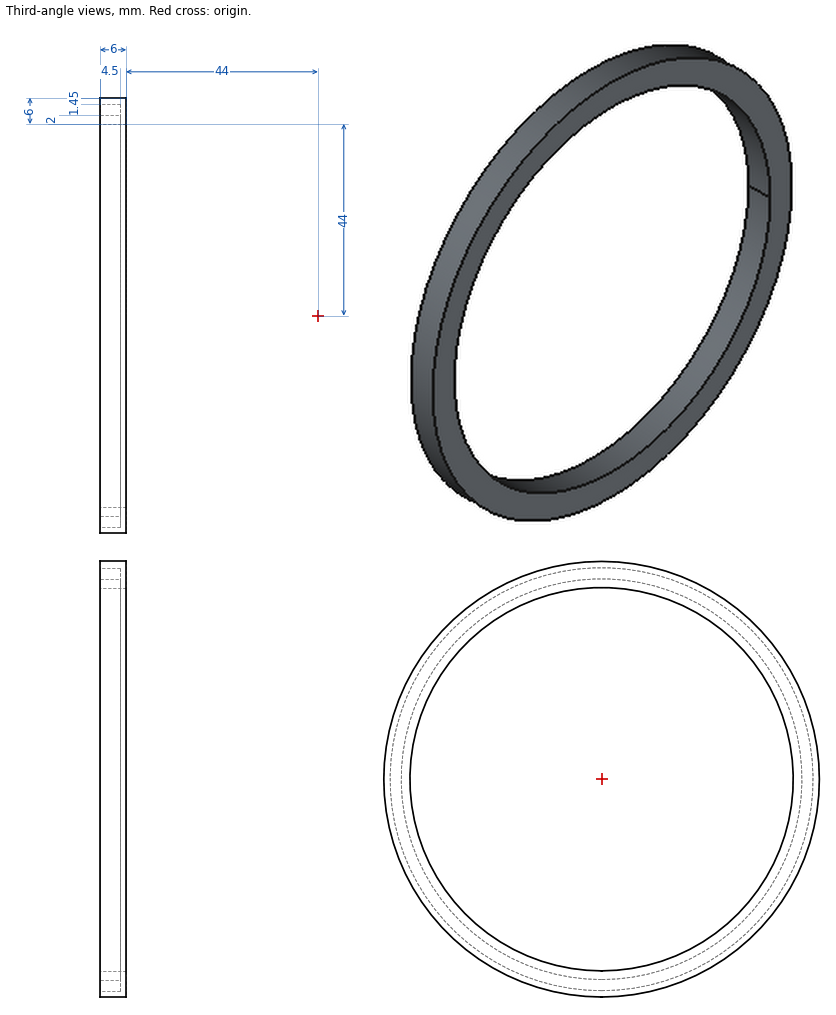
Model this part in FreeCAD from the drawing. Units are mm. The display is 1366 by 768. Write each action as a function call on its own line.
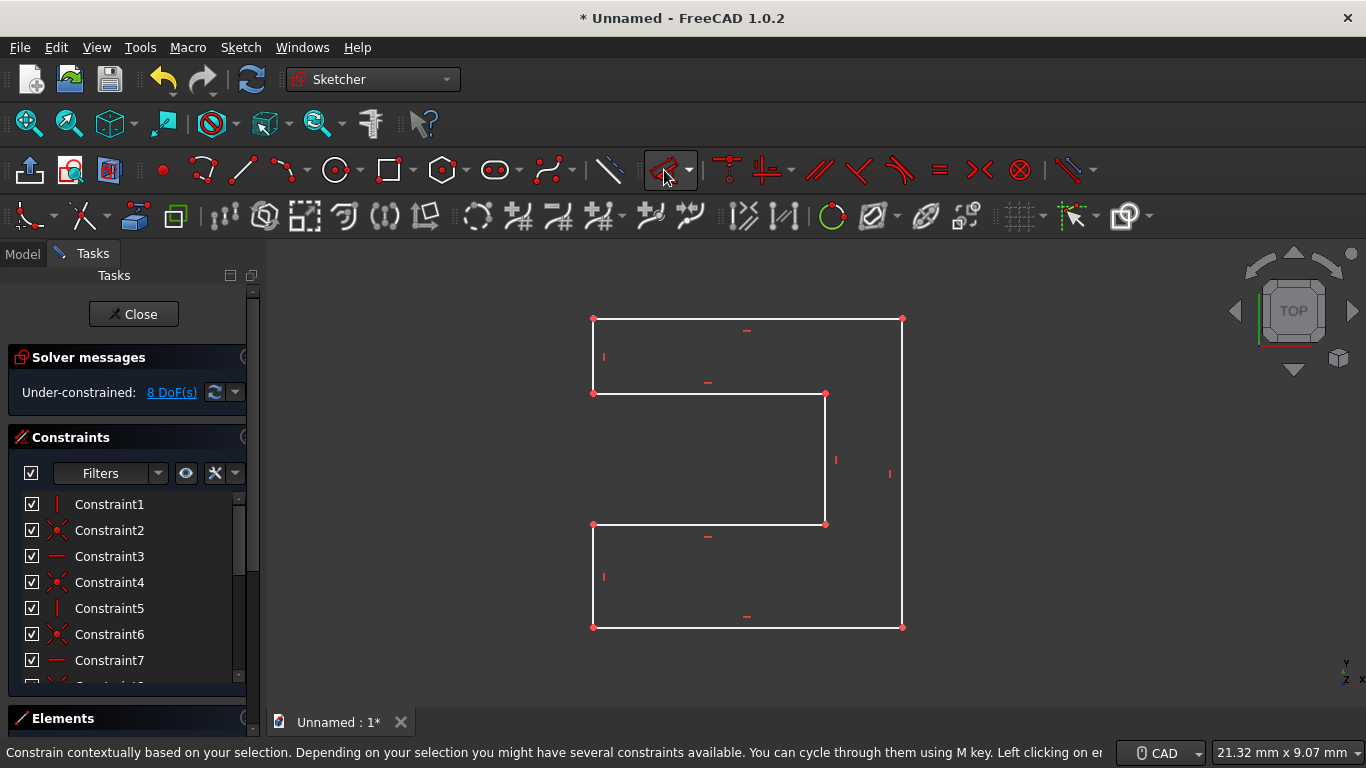
click(902, 535)
click(936, 473)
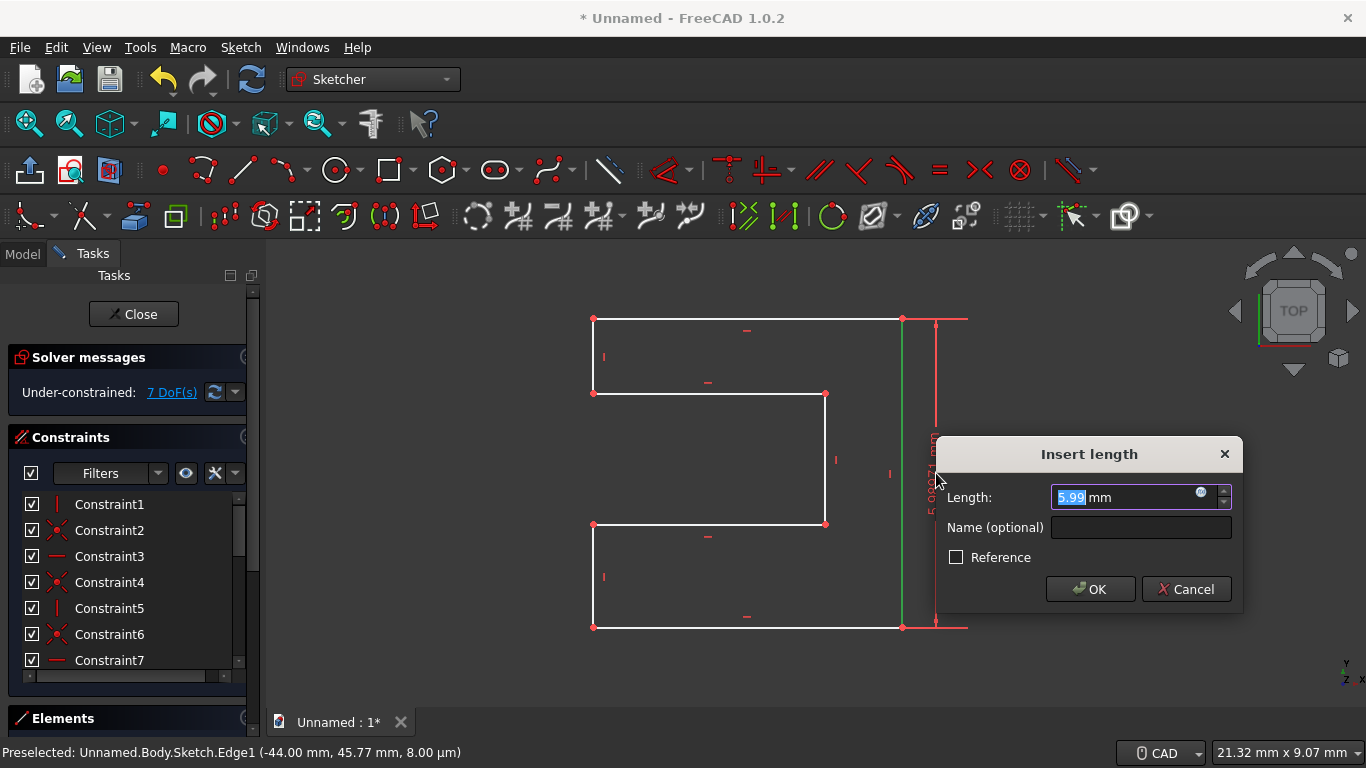
text(6)
key(Return)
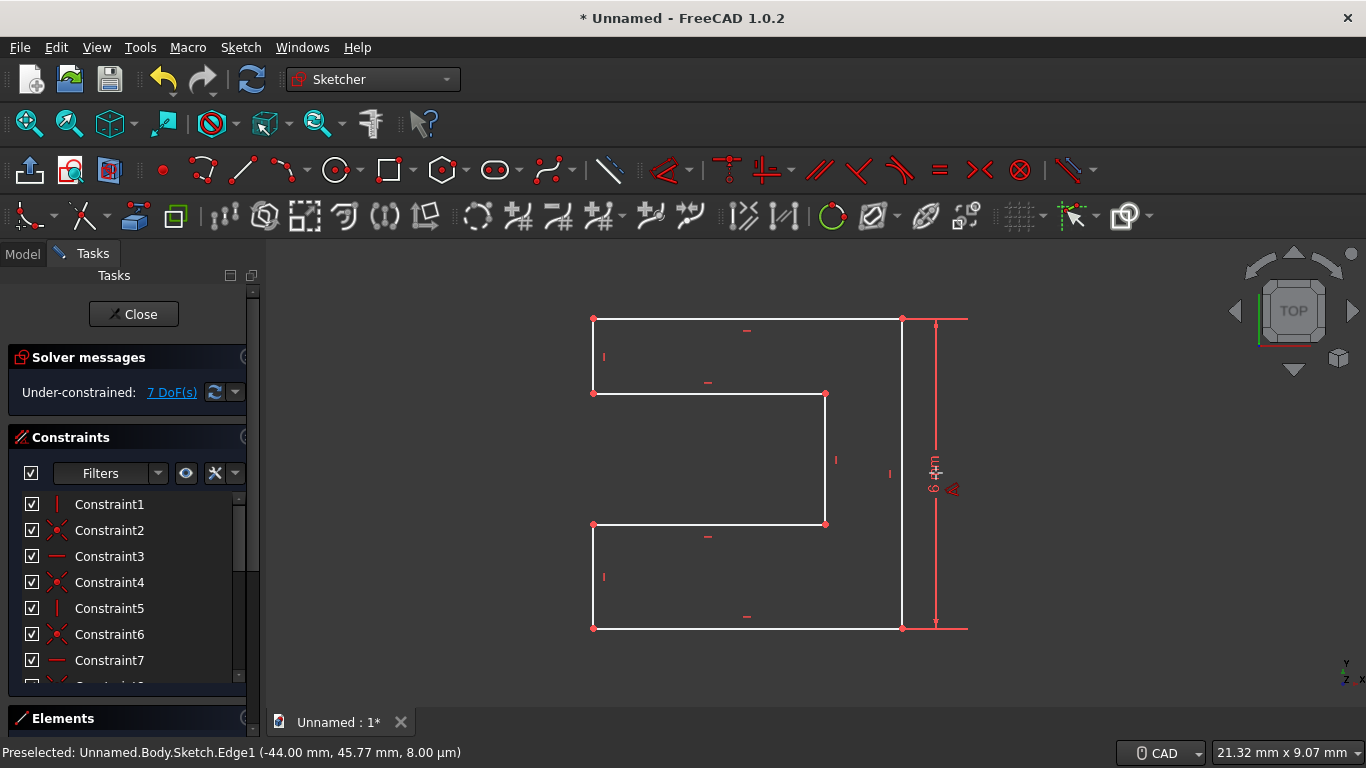
click(809, 319)
click(747, 285)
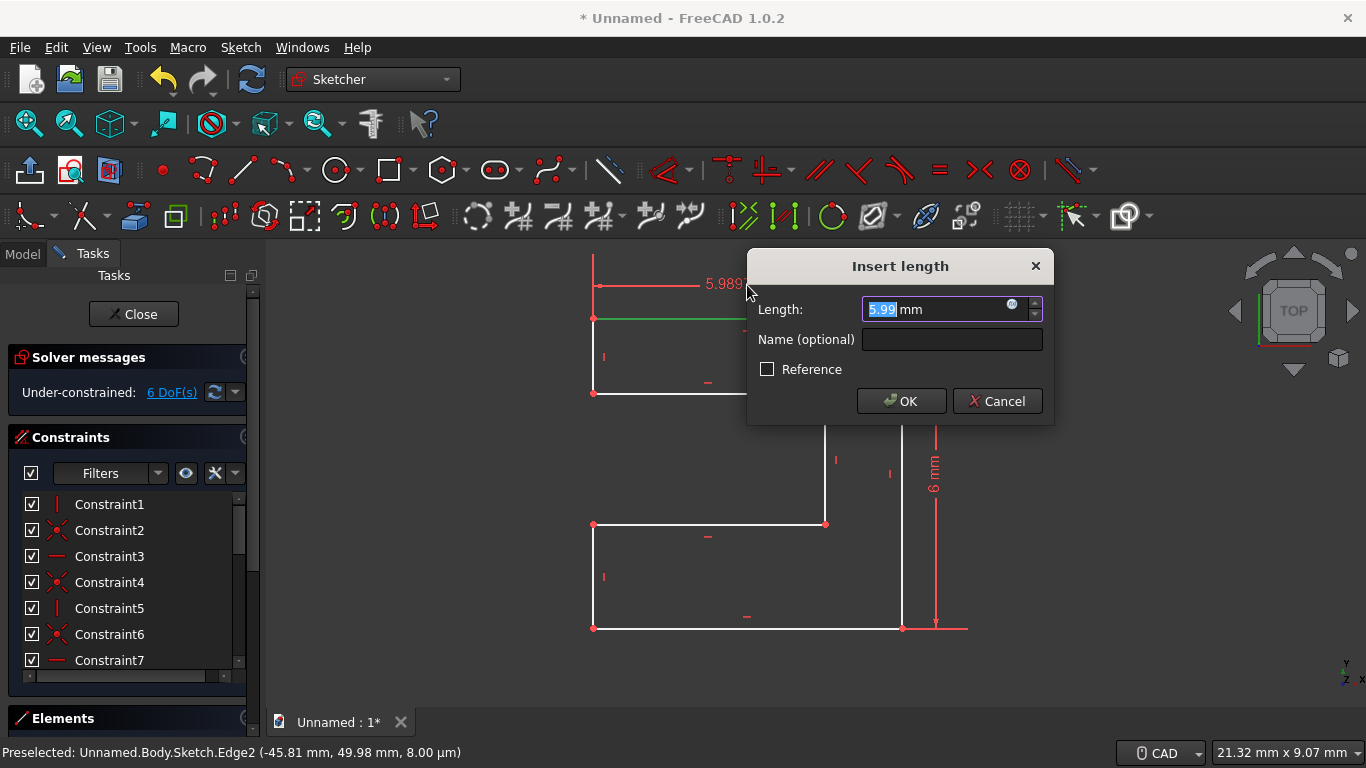
text(6)
key(Return)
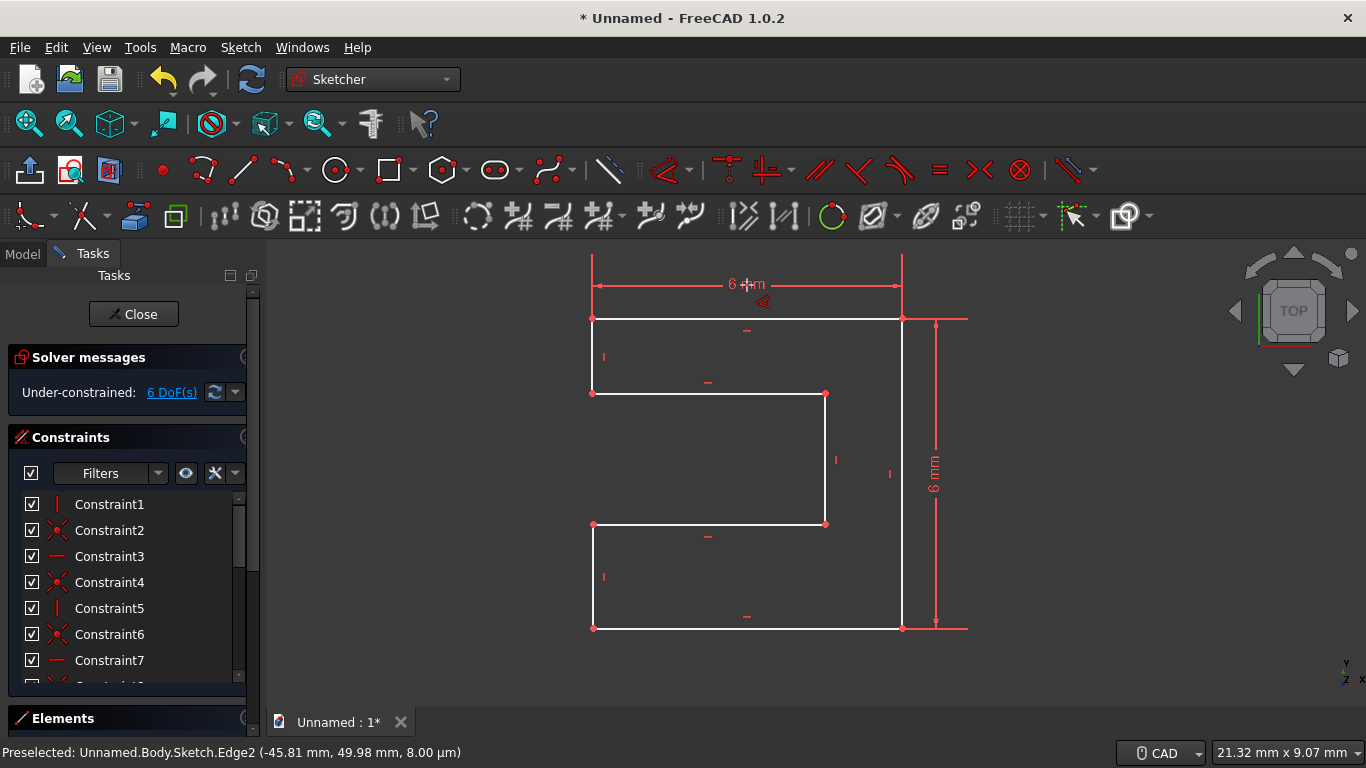
click(593, 556)
click(559, 577)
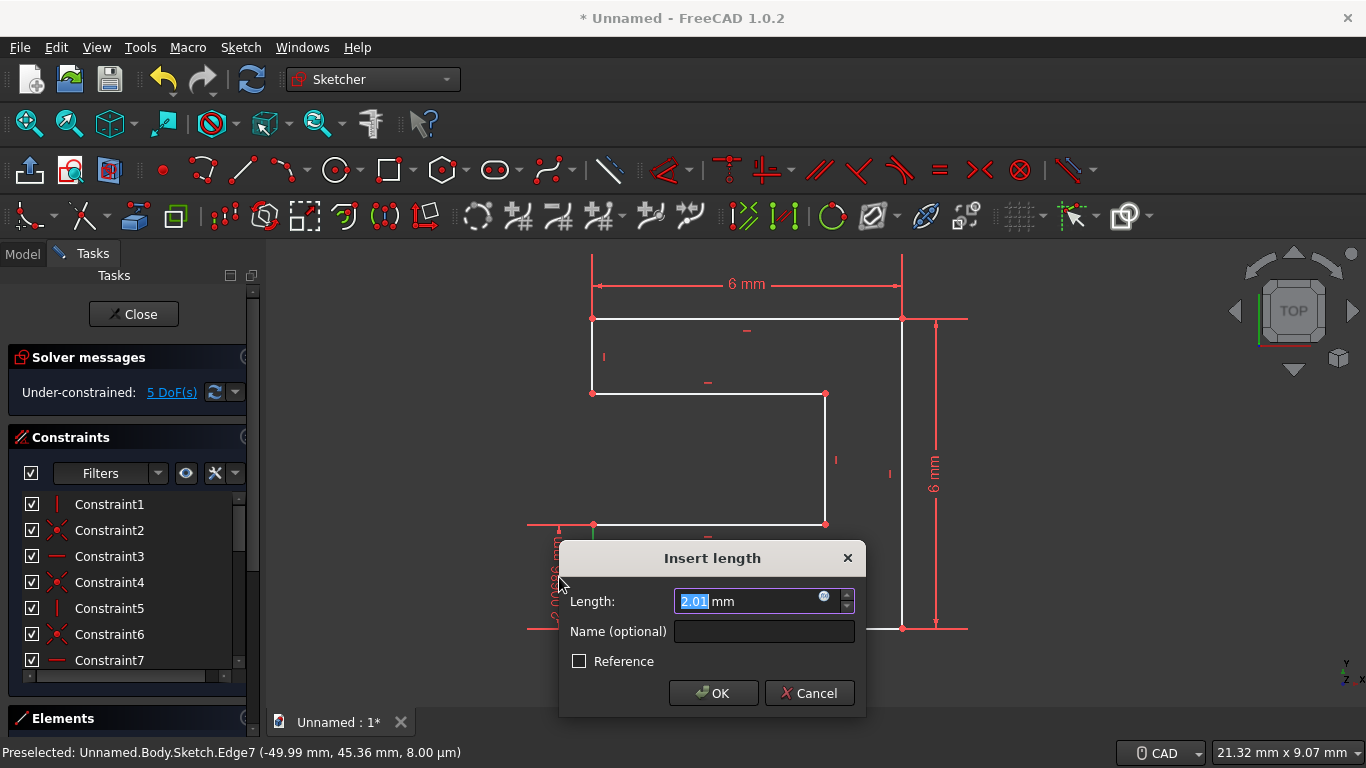
text(2)
key(Return)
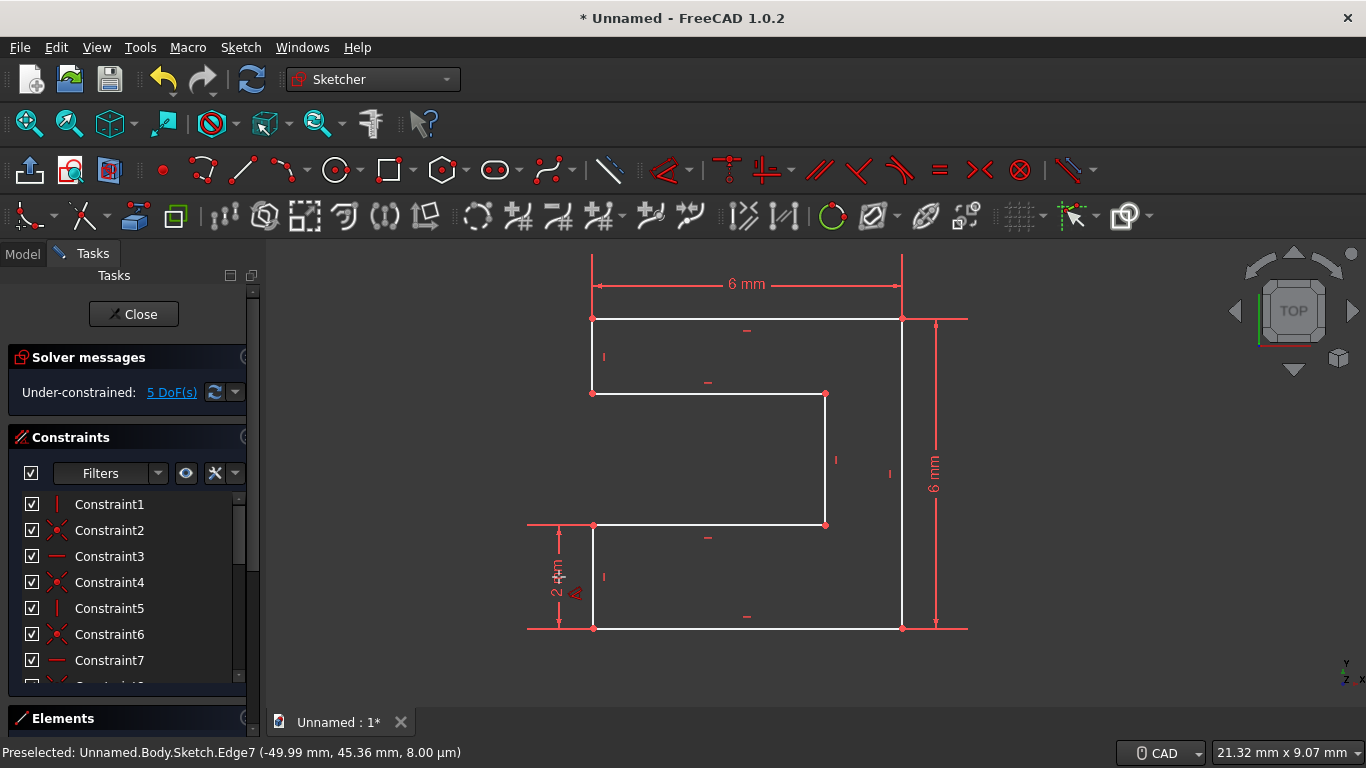
click(686, 629)
click(747, 663)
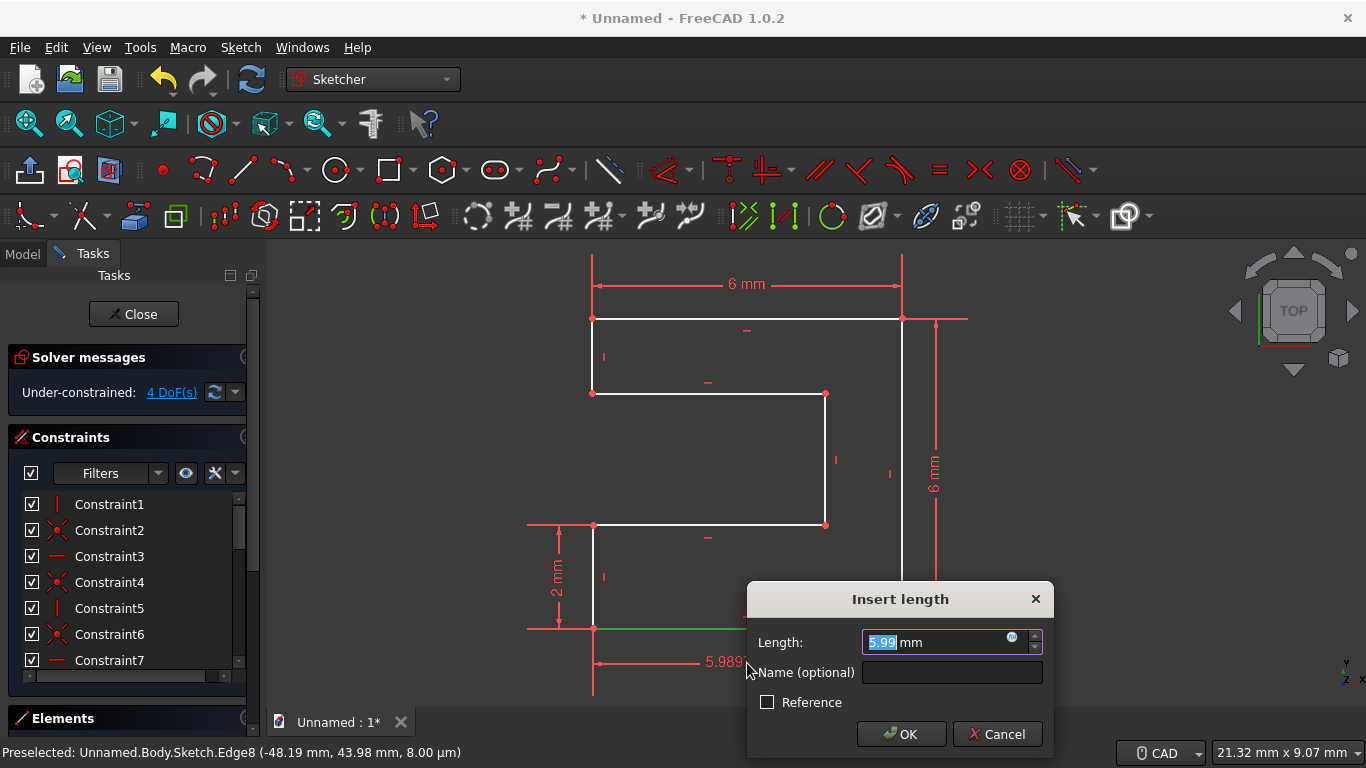
text(6)
key(Return)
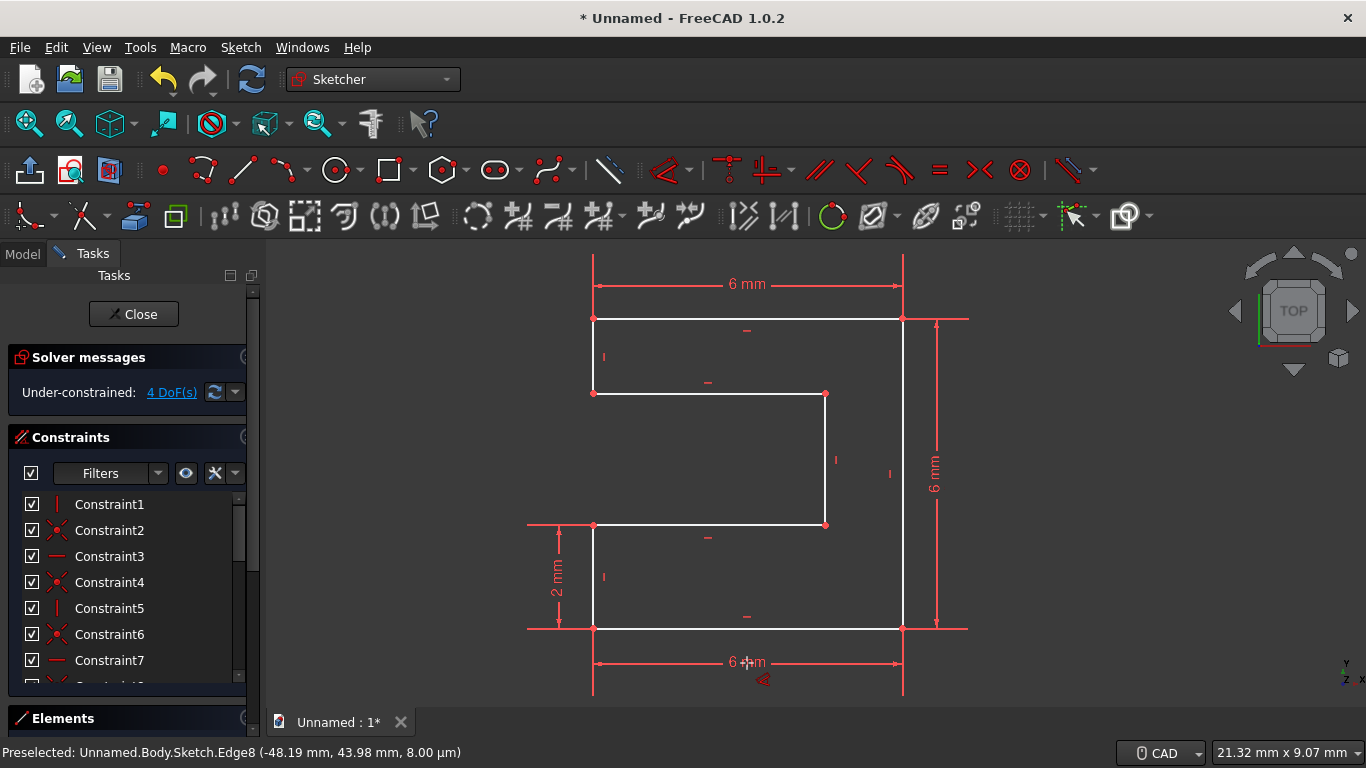
click(663, 394)
click(709, 360)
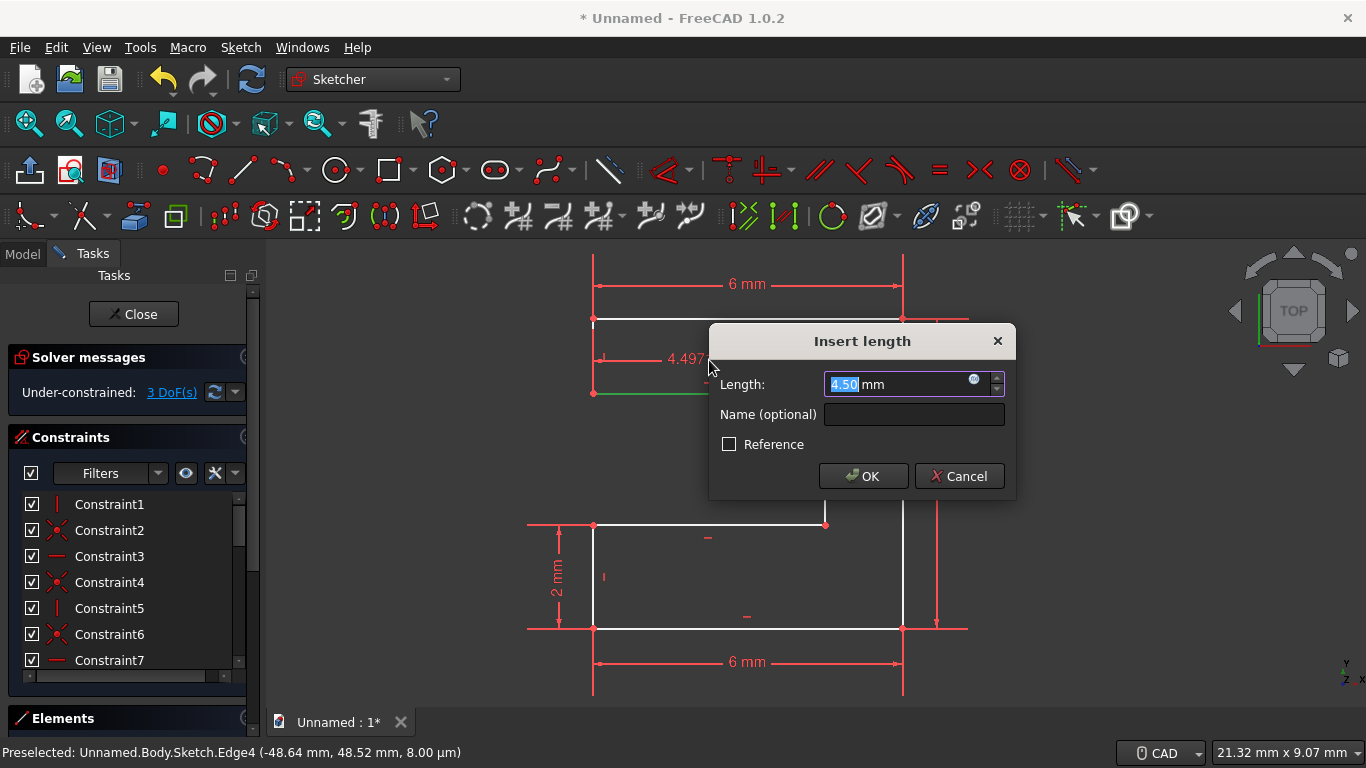
text(4.5)
key(Return)